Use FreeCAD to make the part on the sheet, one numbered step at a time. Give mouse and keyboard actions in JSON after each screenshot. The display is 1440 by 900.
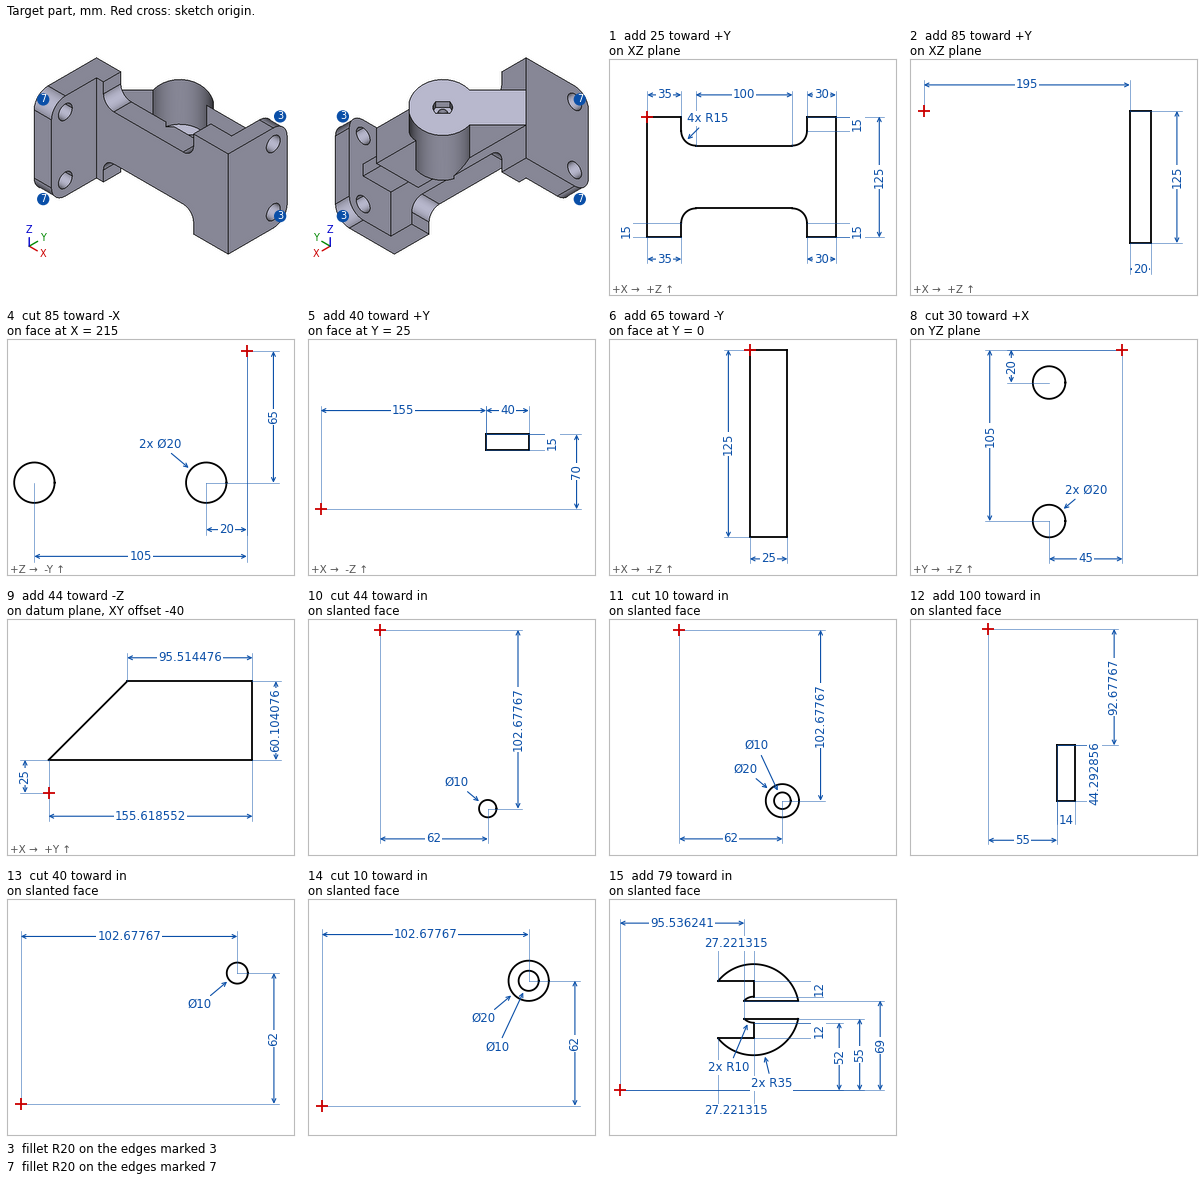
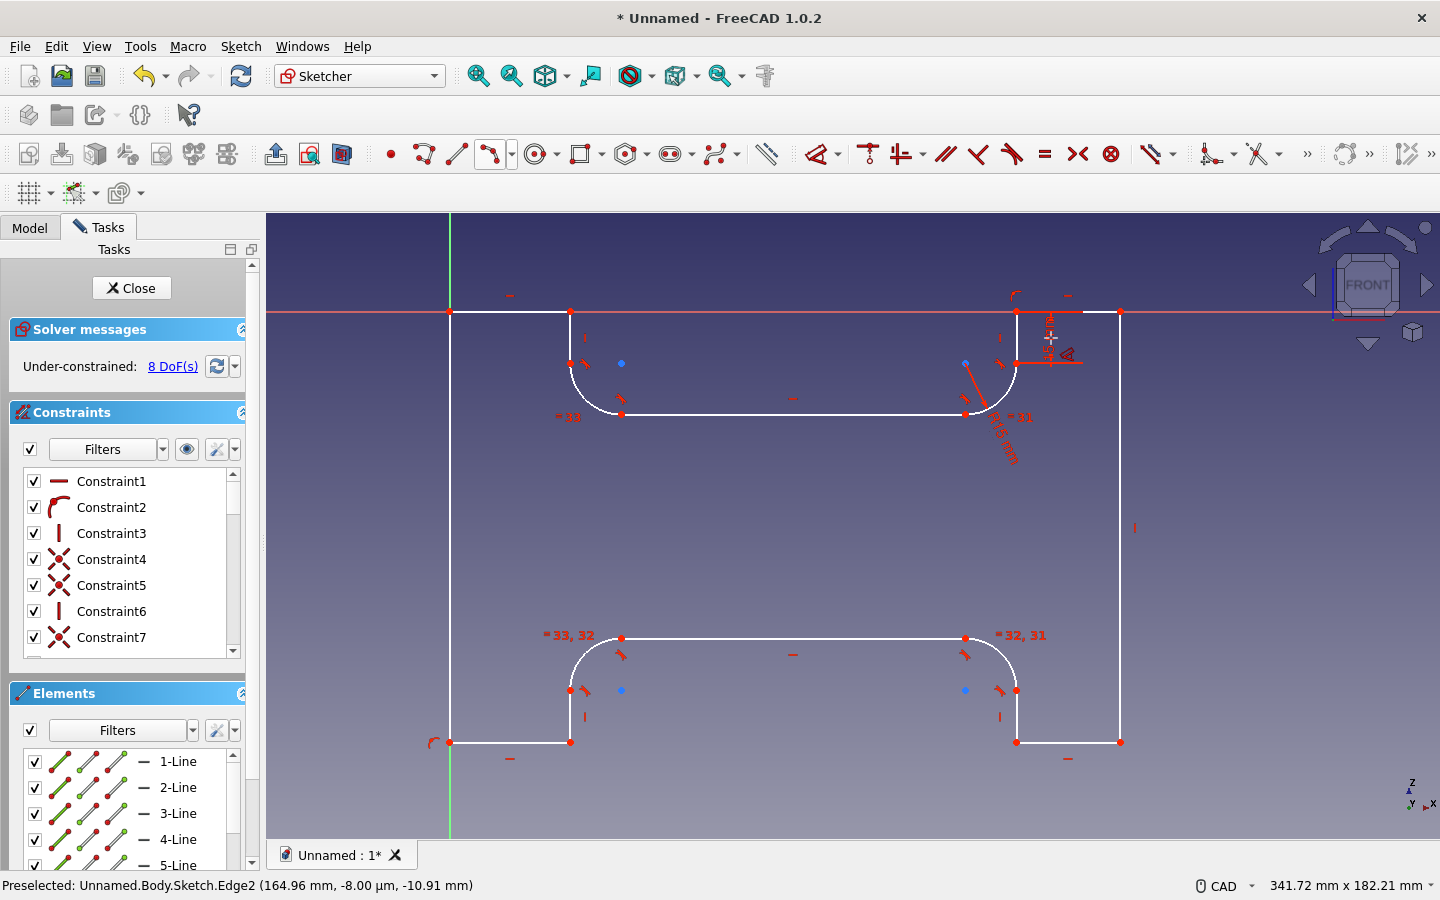
{"action": "left_click", "coordinate": [1048, 312]}
{"action": "left_click", "coordinate": [1068, 278]}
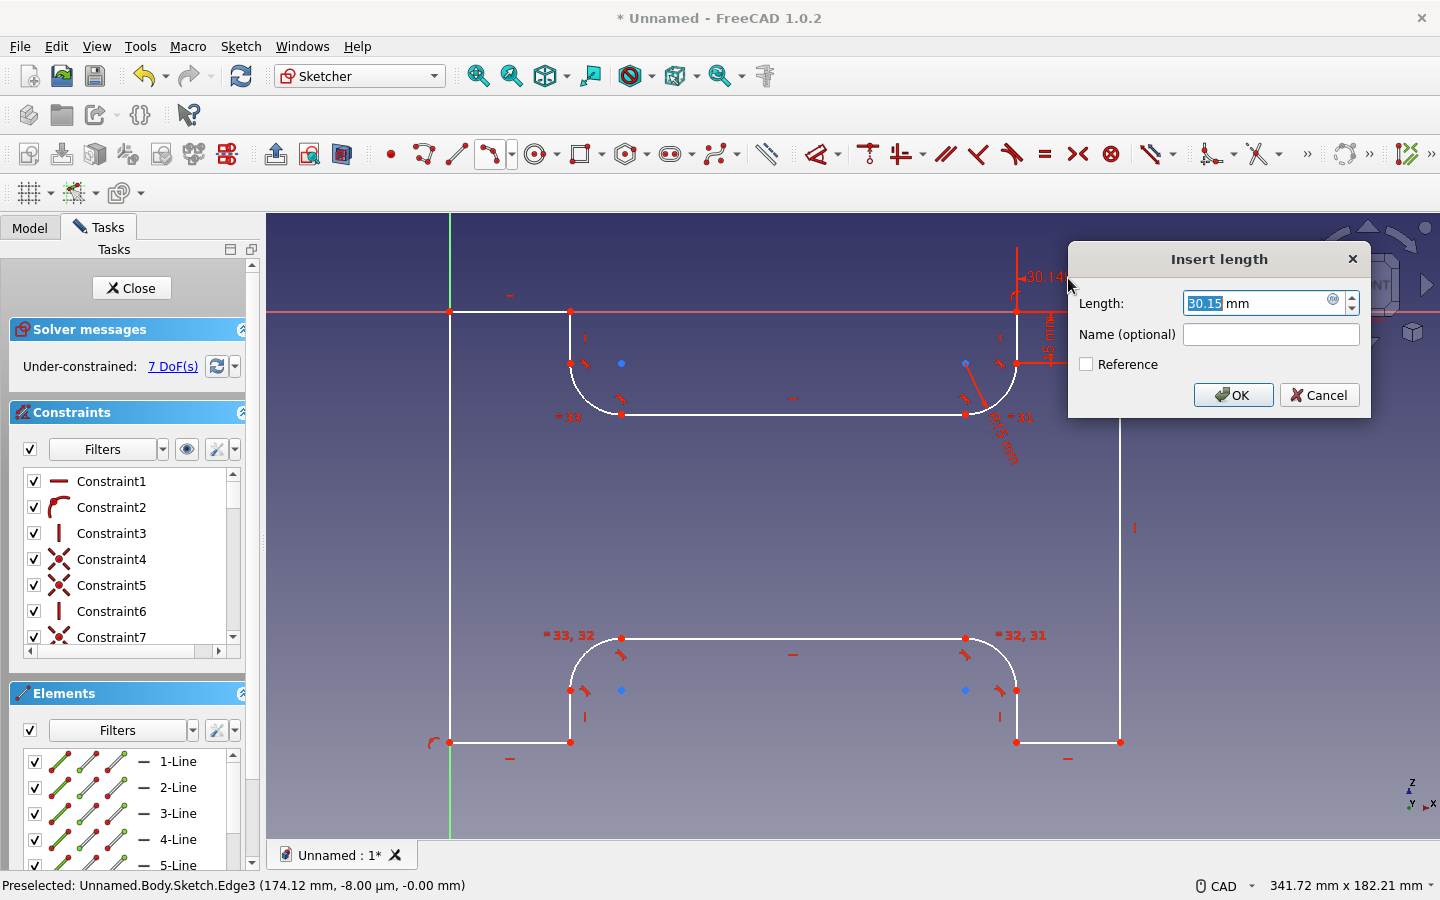
{"action": "type", "text": "30"}
{"action": "key", "text": "Return"}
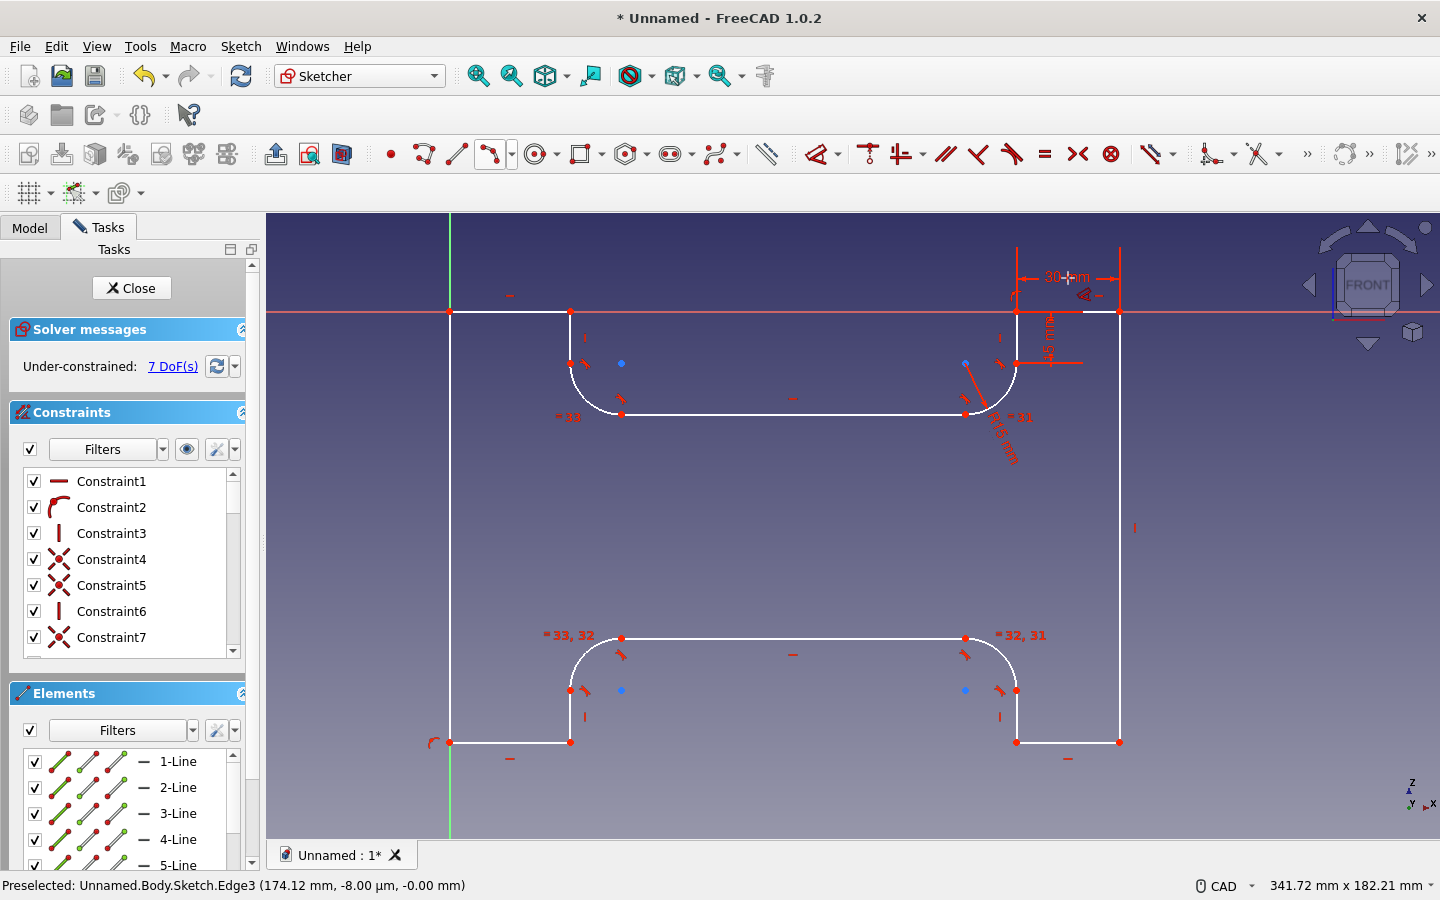
{"action": "left_click", "coordinate": [1089, 743]}
{"action": "left_click", "coordinate": [1068, 777]}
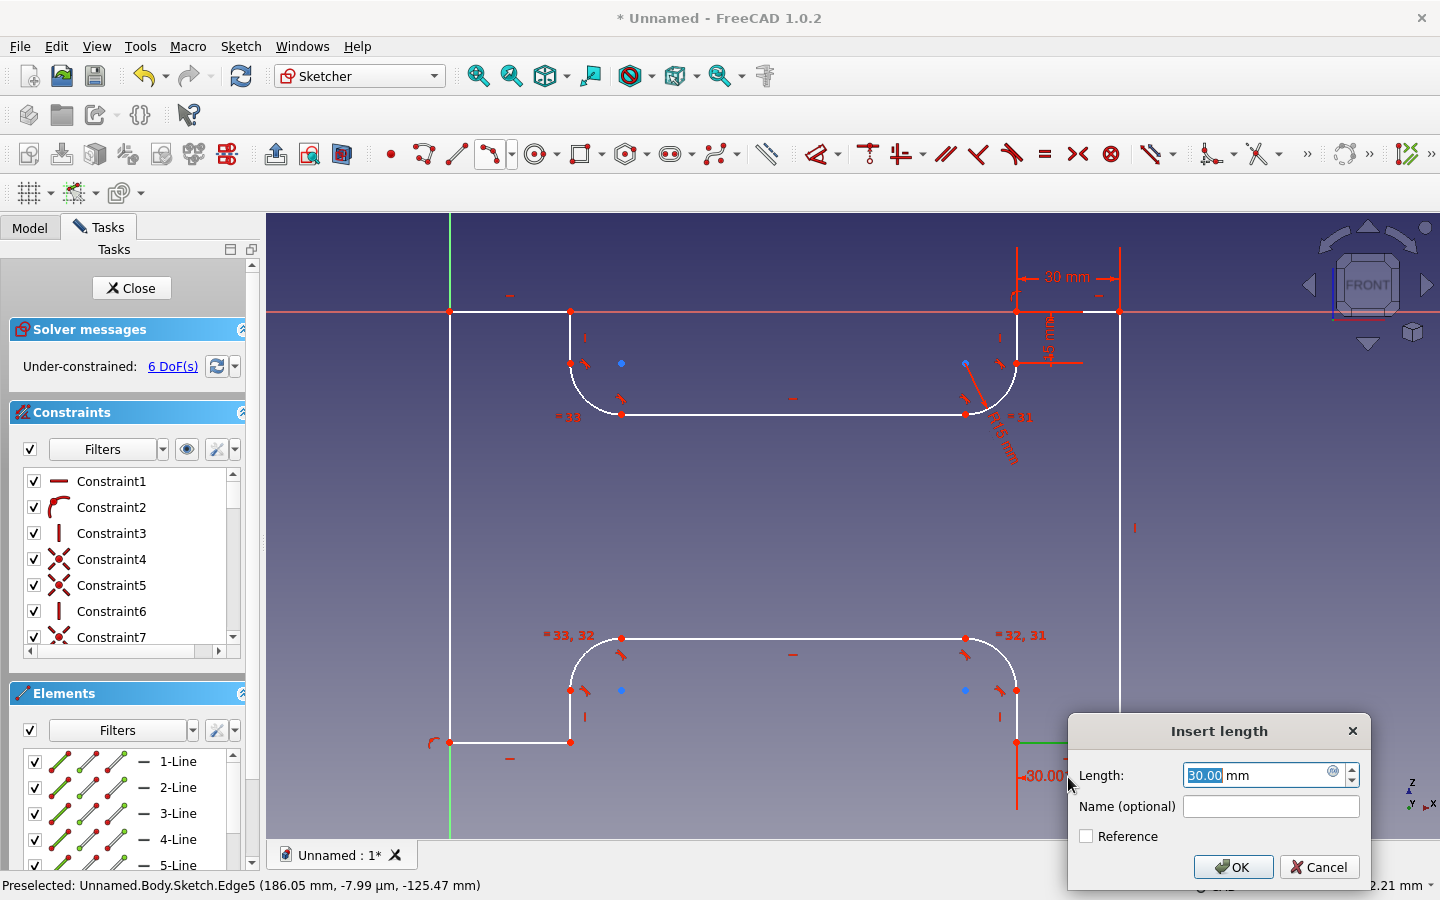
{"action": "type", "text": "30"}
{"action": "key", "text": "Return"}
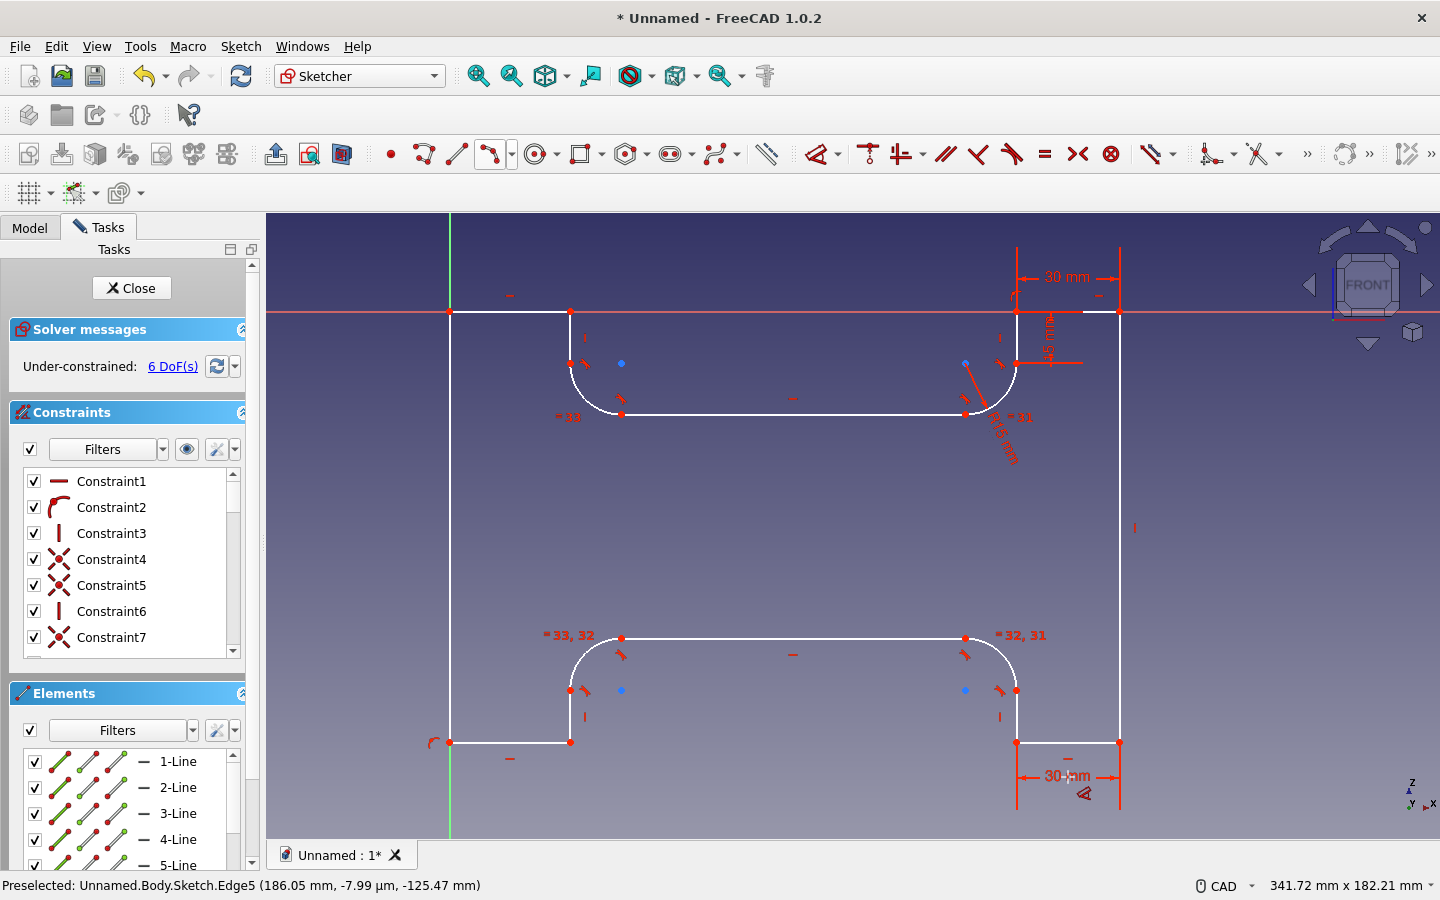
{"action": "left_click", "coordinate": [1017, 727]}
{"action": "left_click", "coordinate": [1051, 716]}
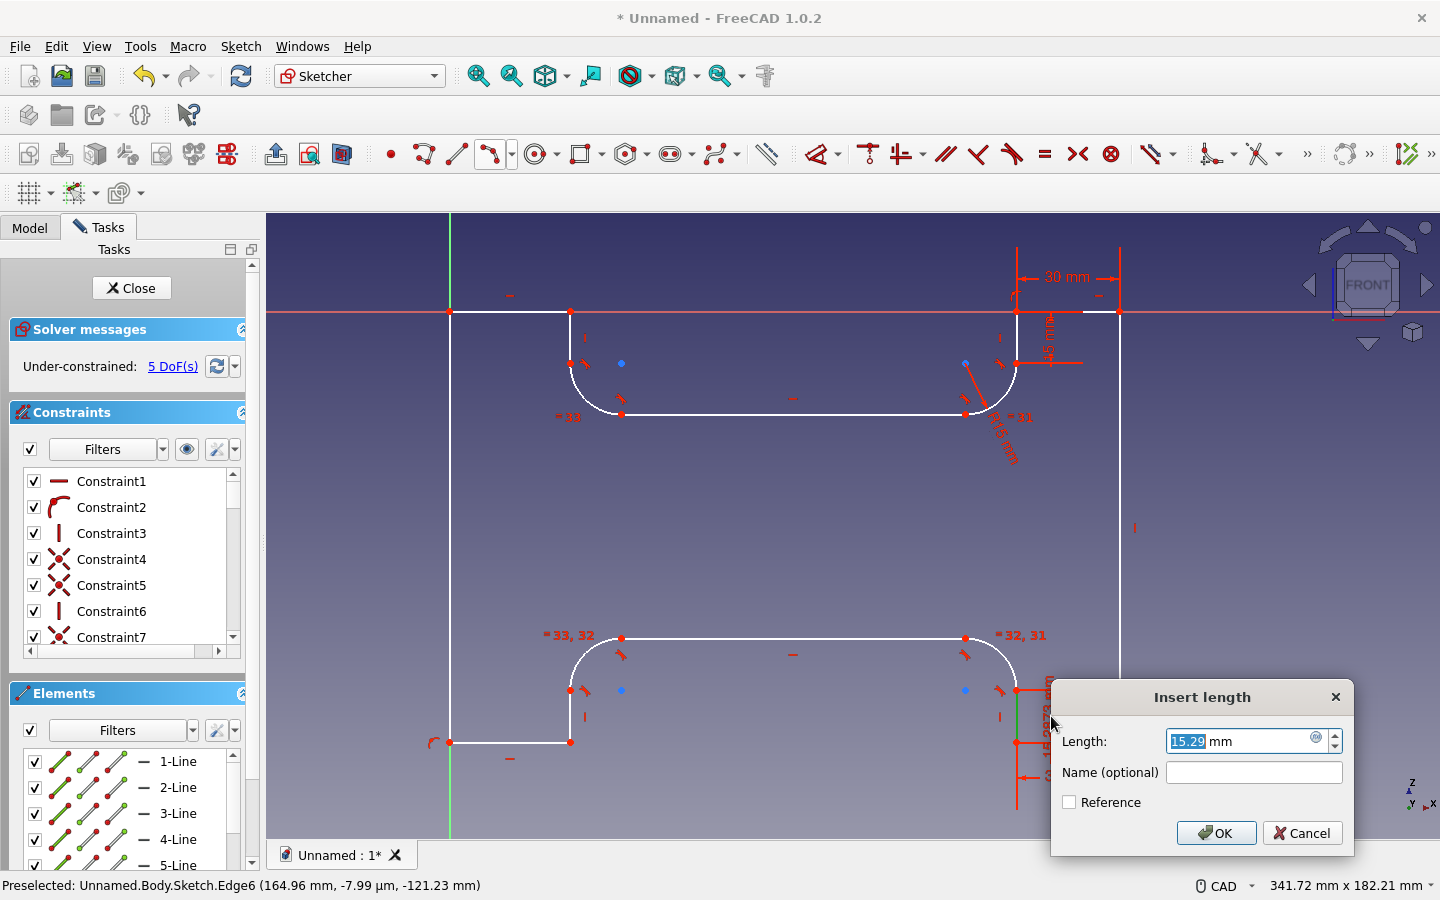
{"action": "type", "text": "15"}
{"action": "key", "text": "Return"}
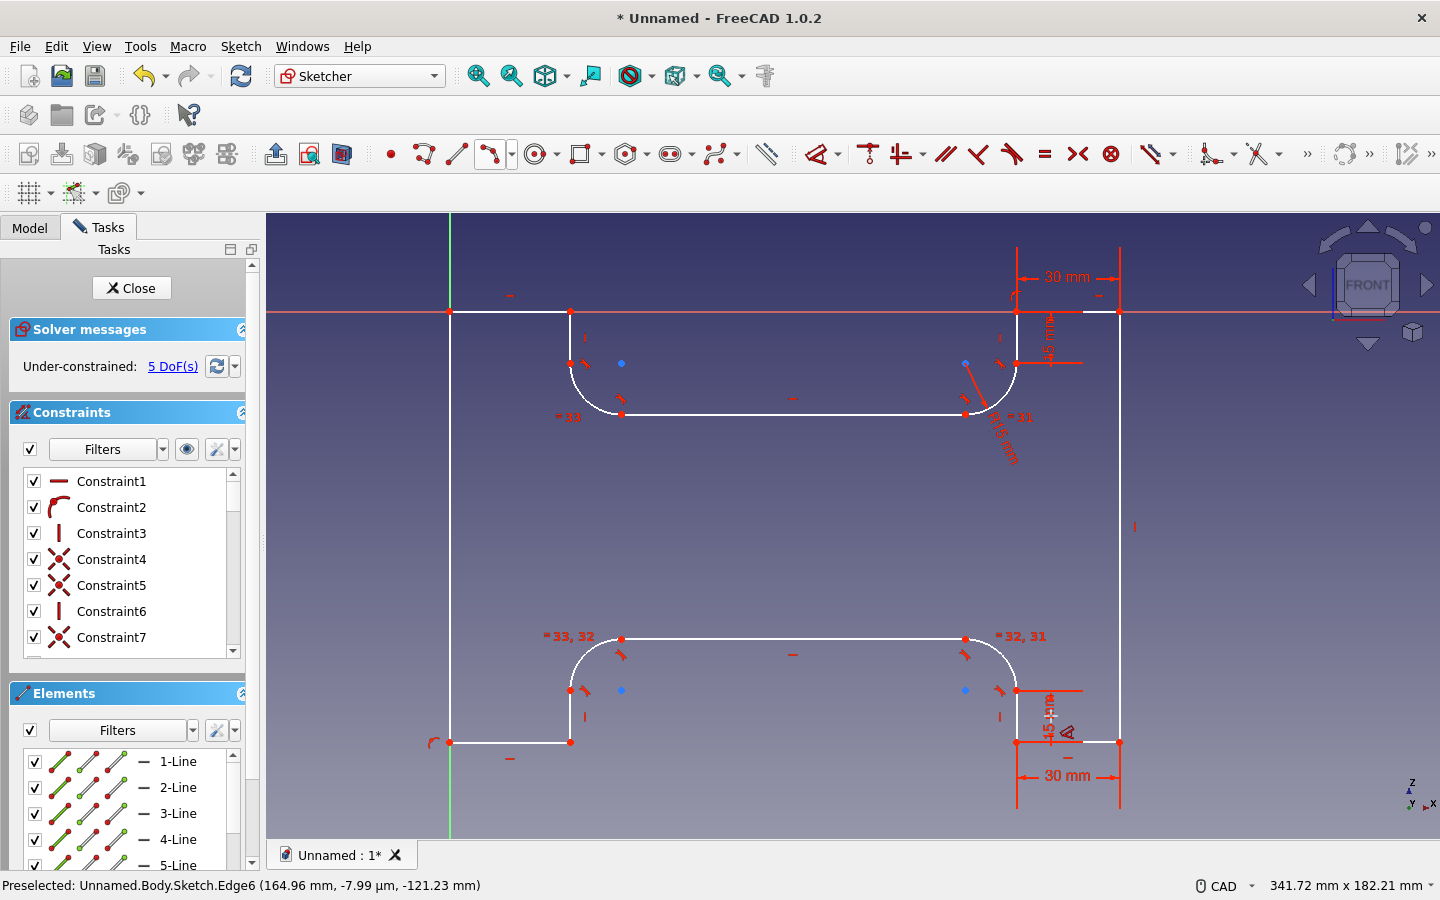
{"action": "left_click", "coordinate": [570, 706]}
{"action": "left_click", "coordinate": [536, 717]}